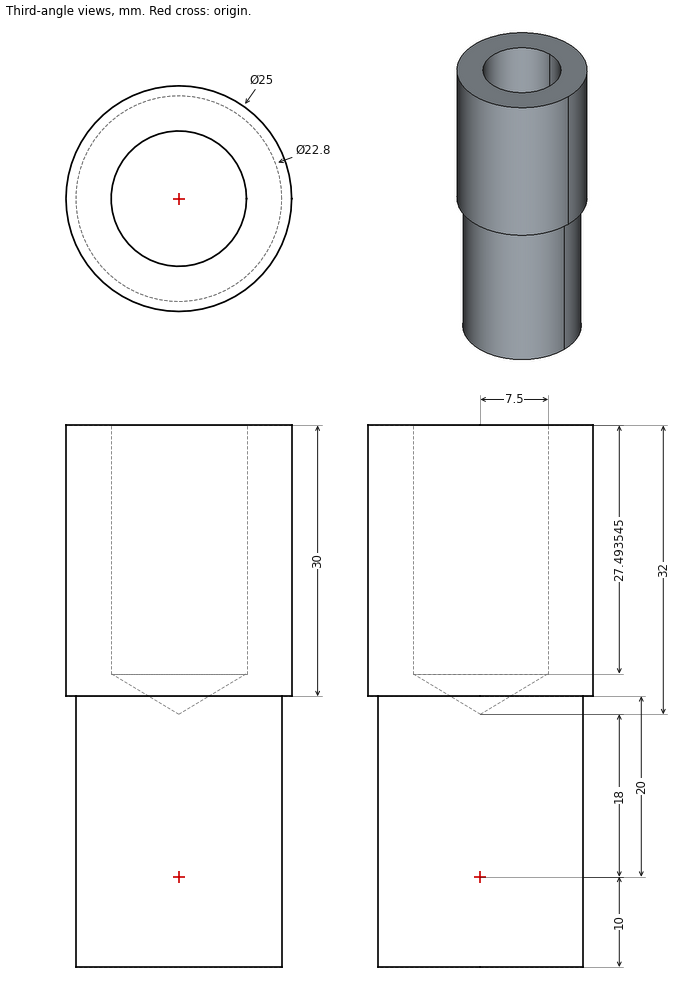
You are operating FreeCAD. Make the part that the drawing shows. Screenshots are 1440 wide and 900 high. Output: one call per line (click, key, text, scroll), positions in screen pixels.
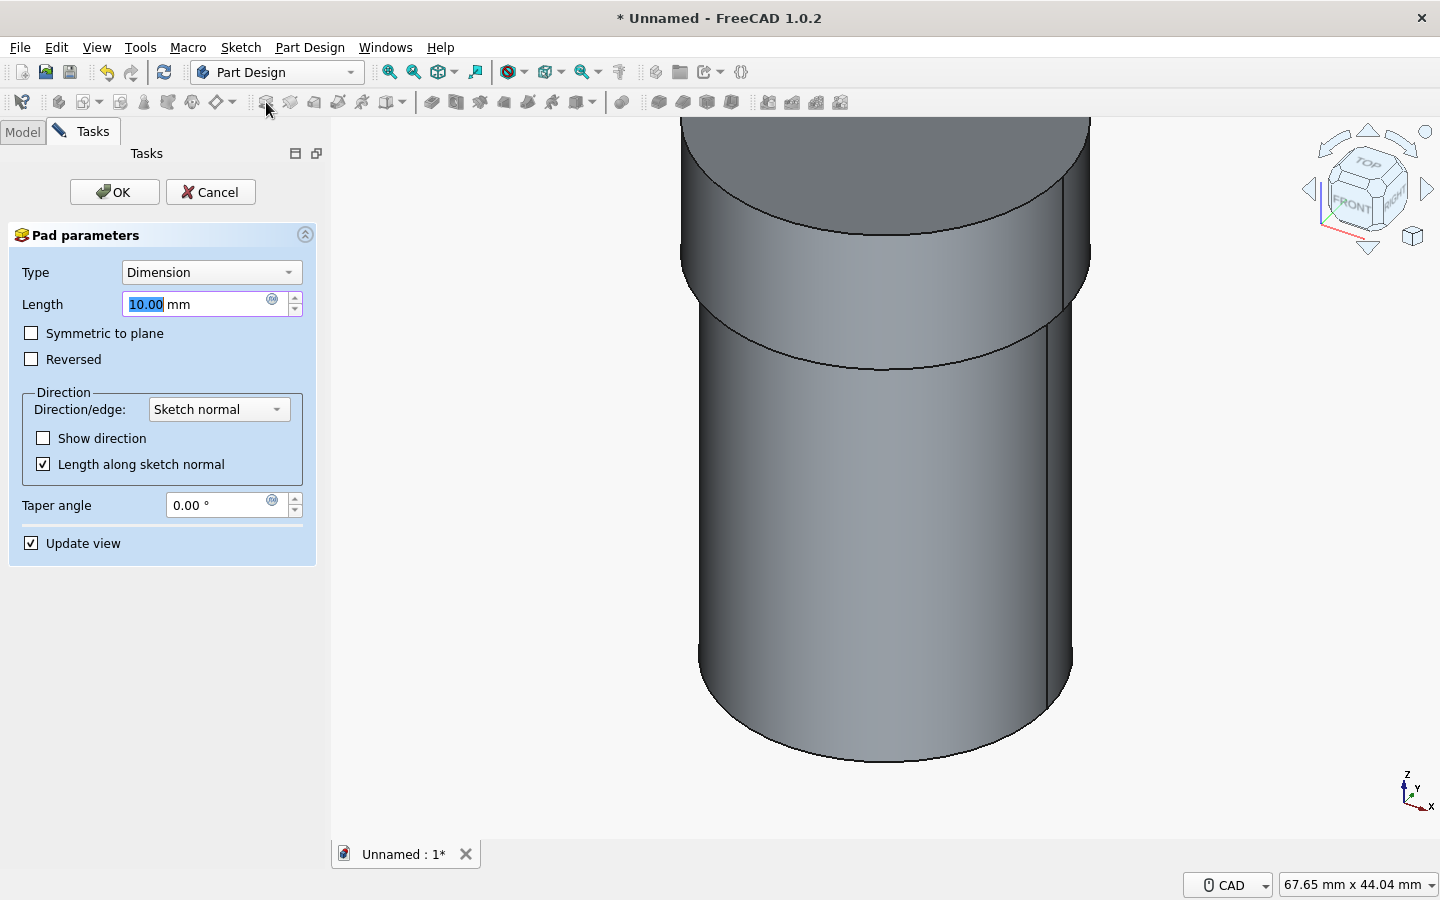
text(30)
key(Tab)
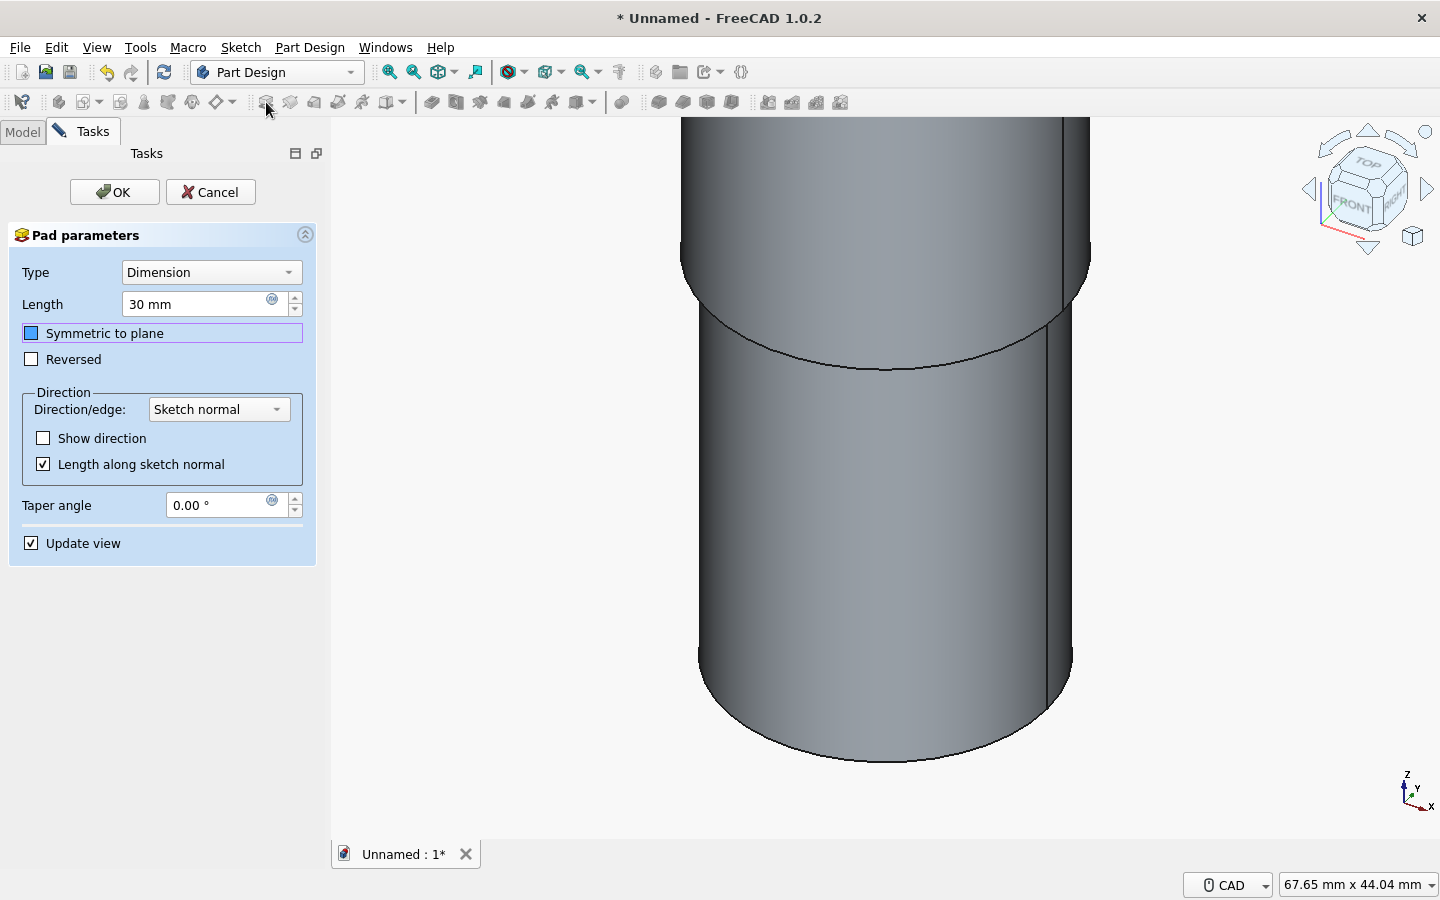
click(115, 192)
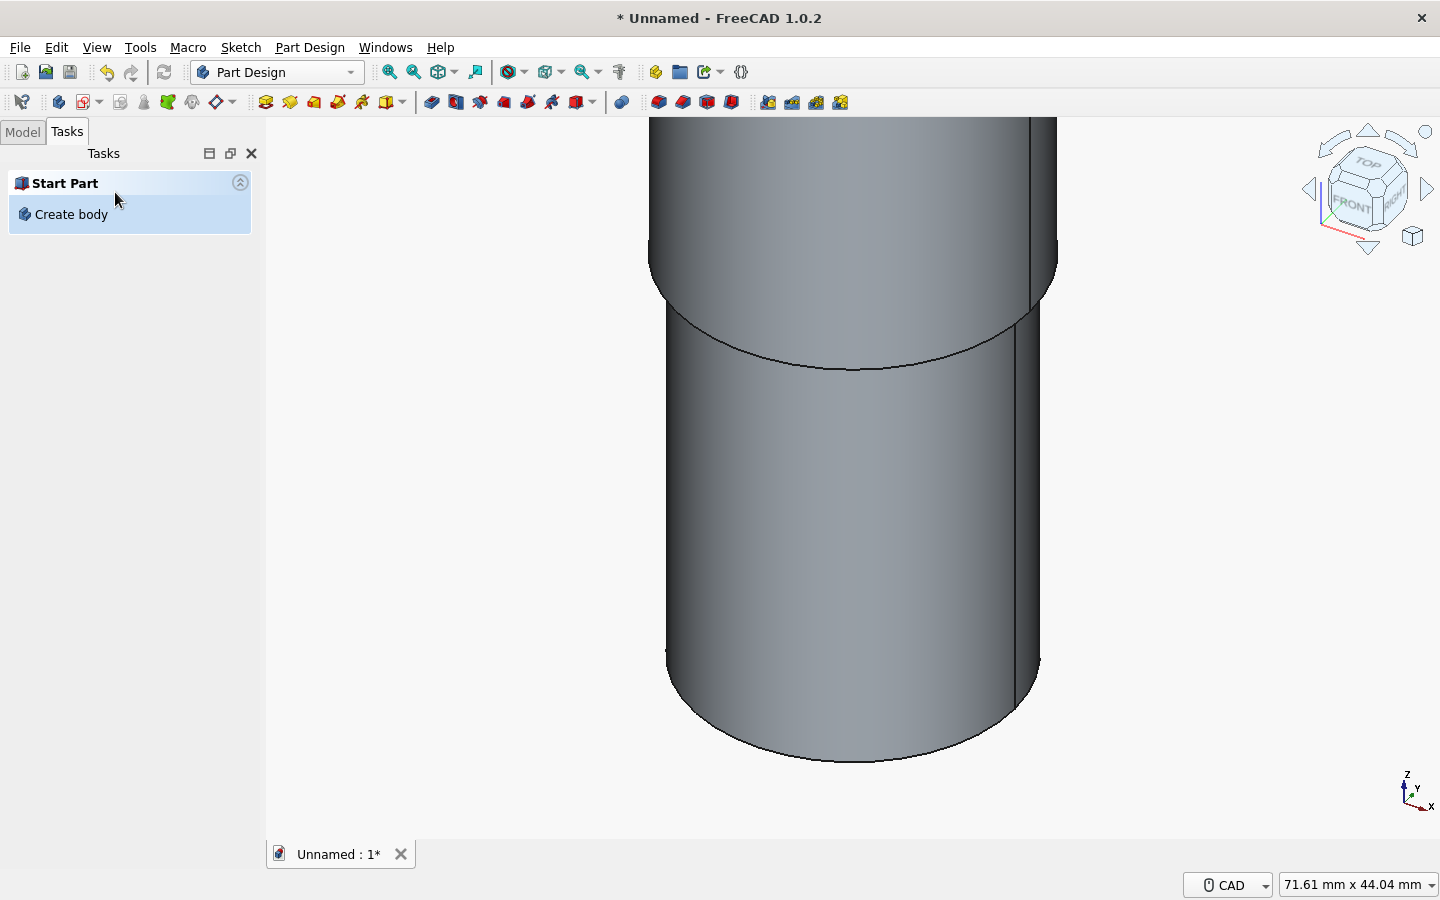
click(390, 72)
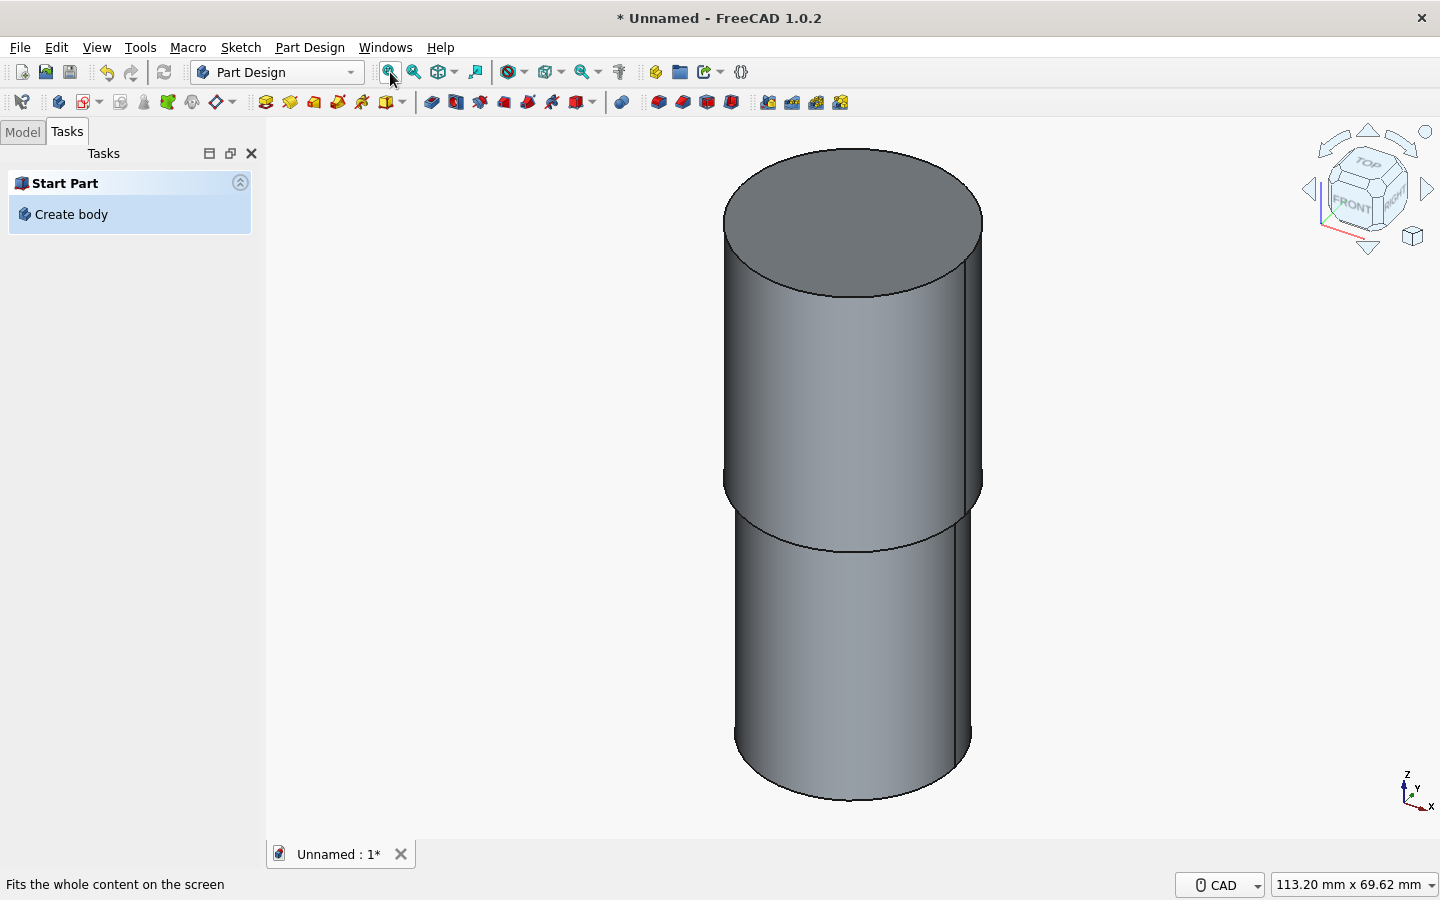
click(84, 102)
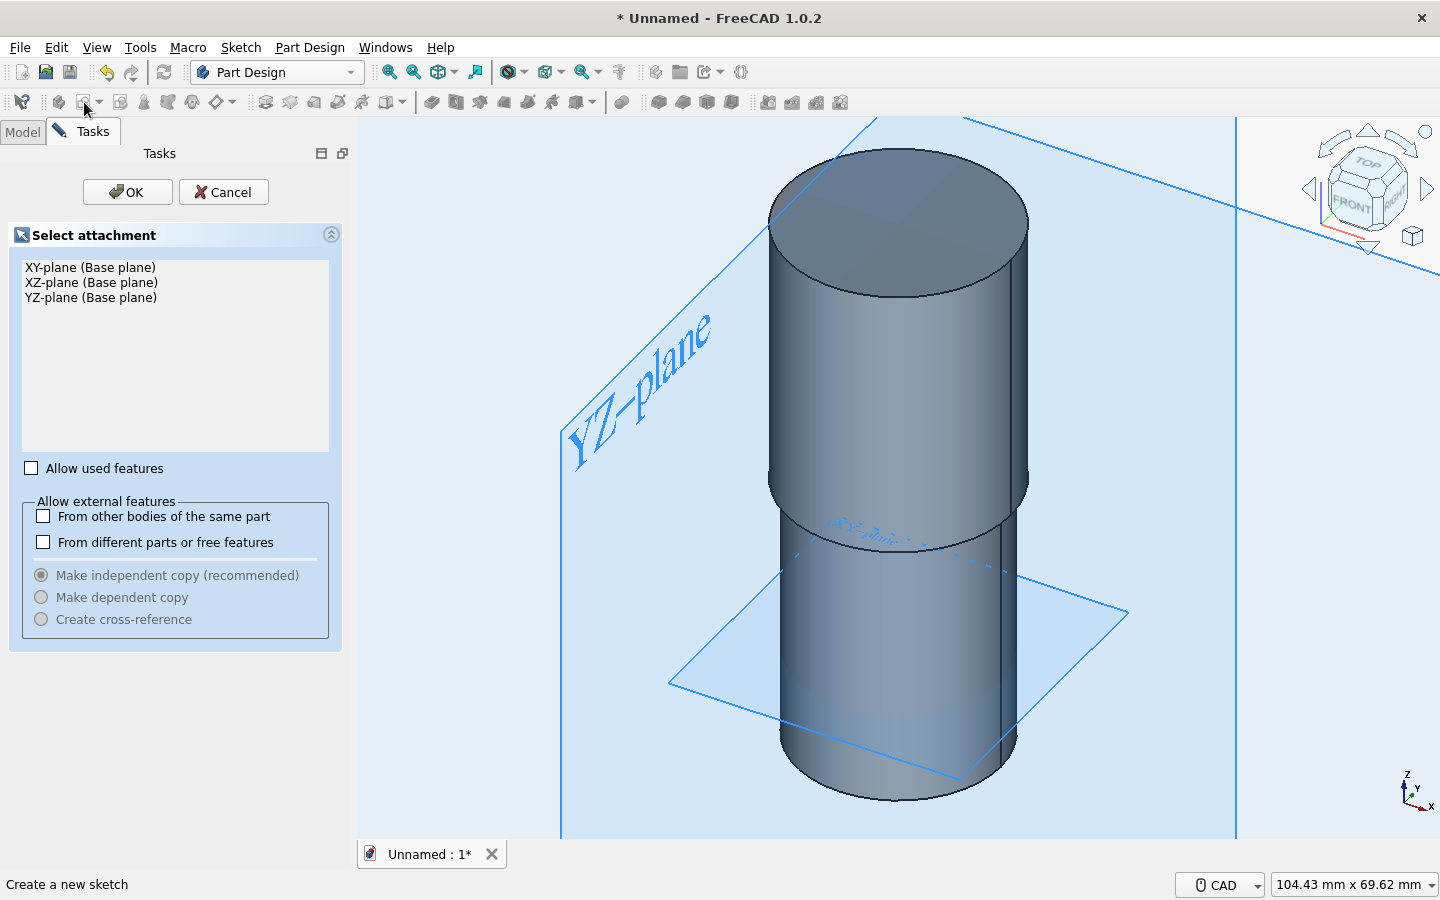
click(82, 298)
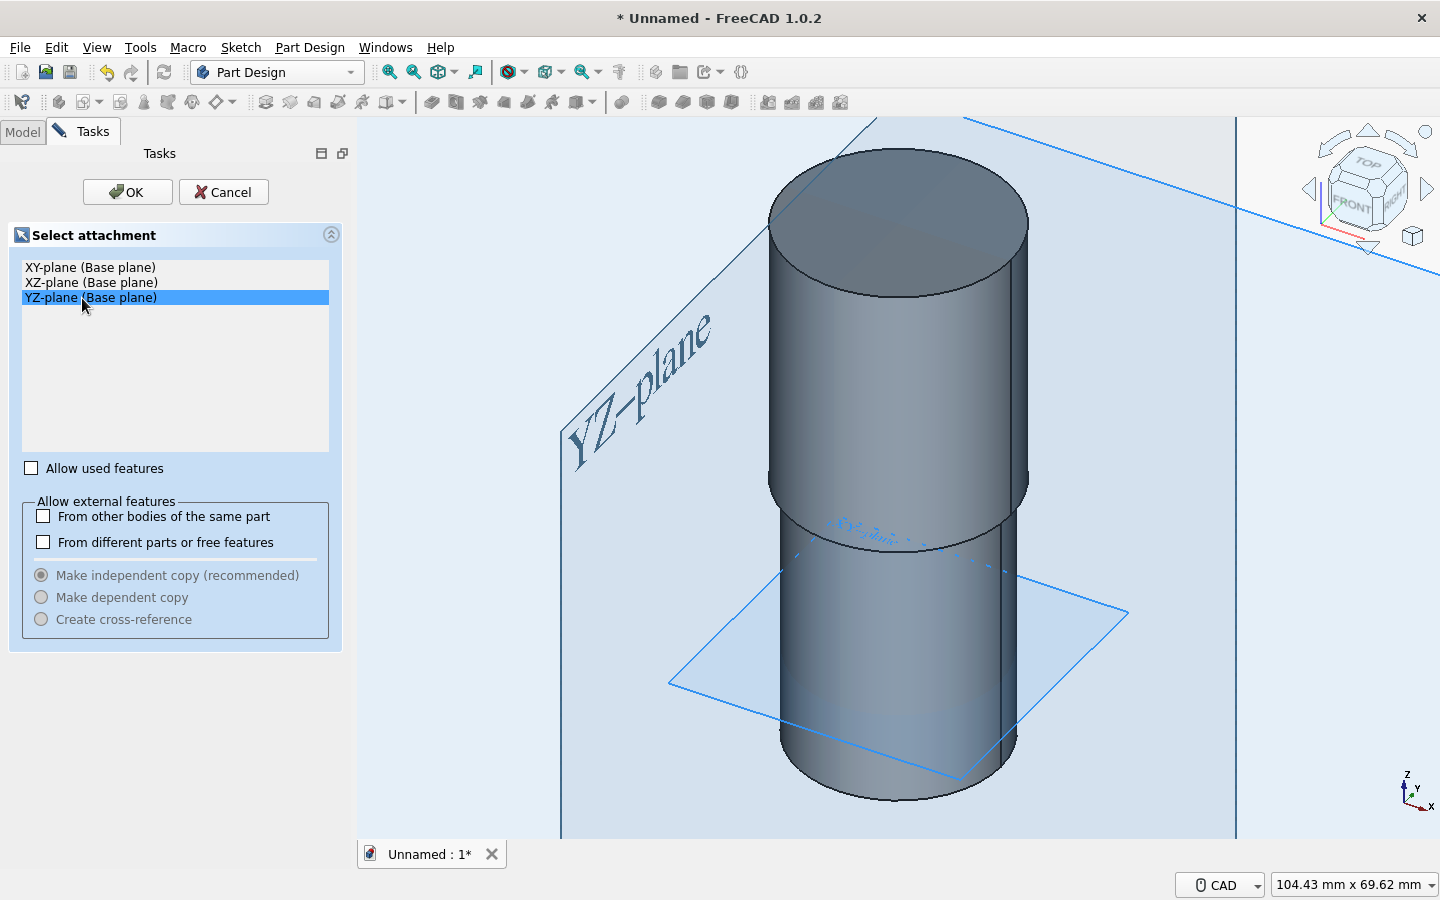
click(128, 192)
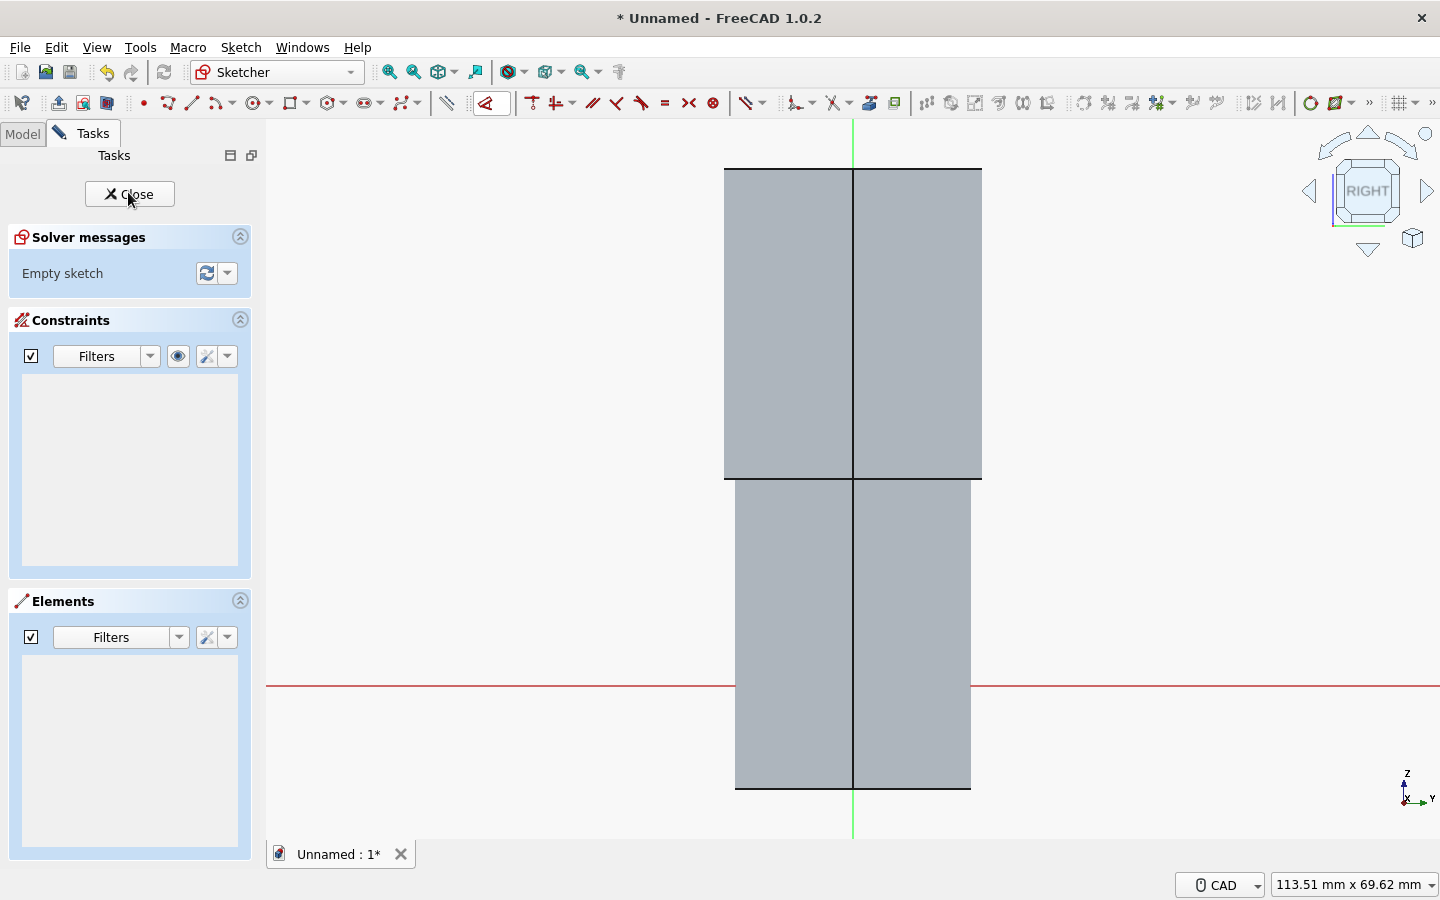
click(108, 104)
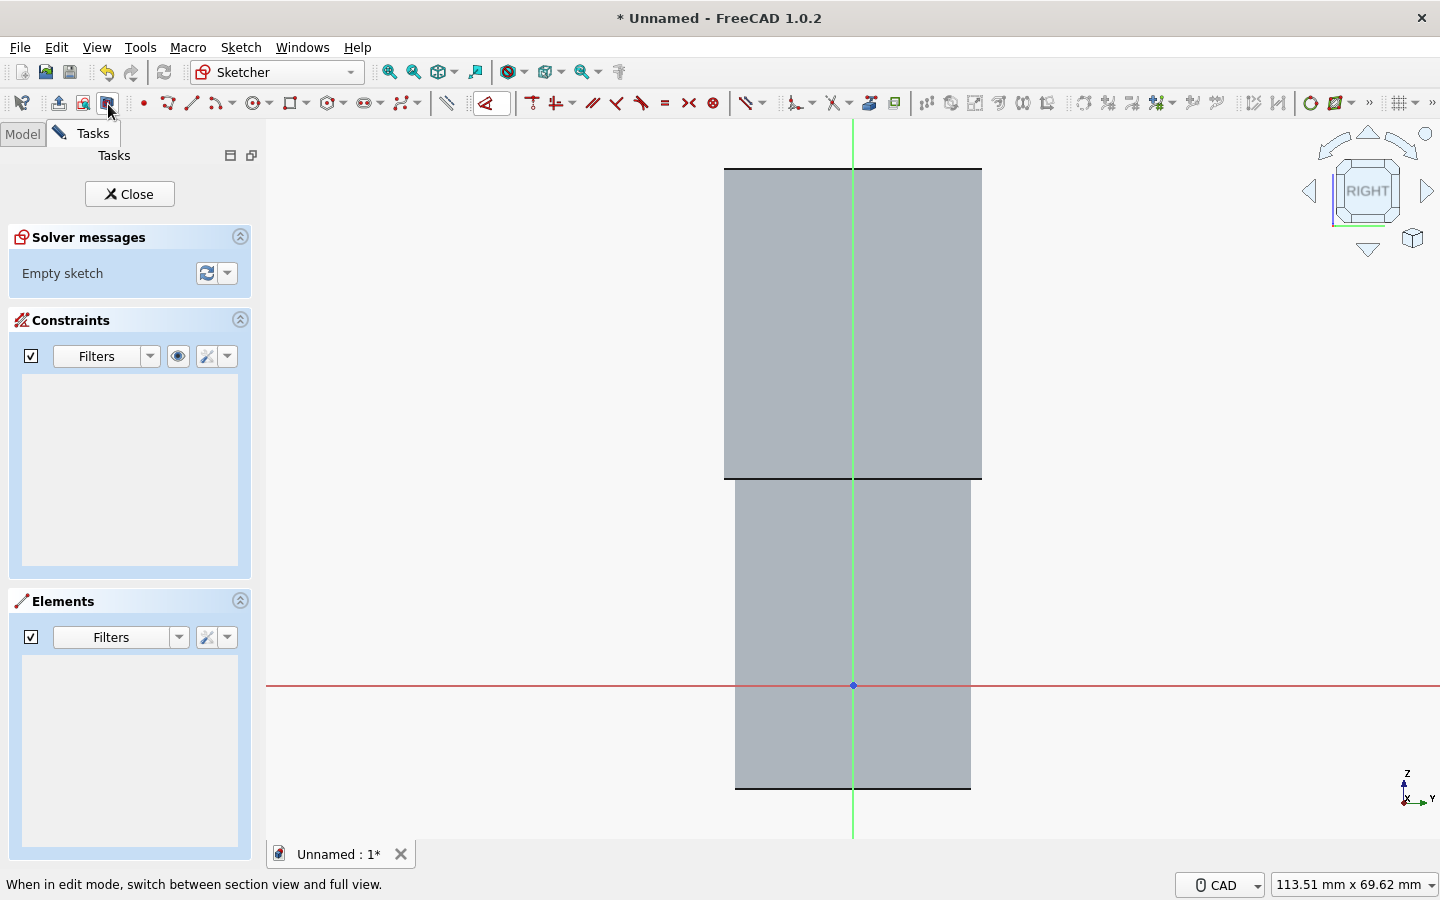
scroll(300, 713, down, 1)